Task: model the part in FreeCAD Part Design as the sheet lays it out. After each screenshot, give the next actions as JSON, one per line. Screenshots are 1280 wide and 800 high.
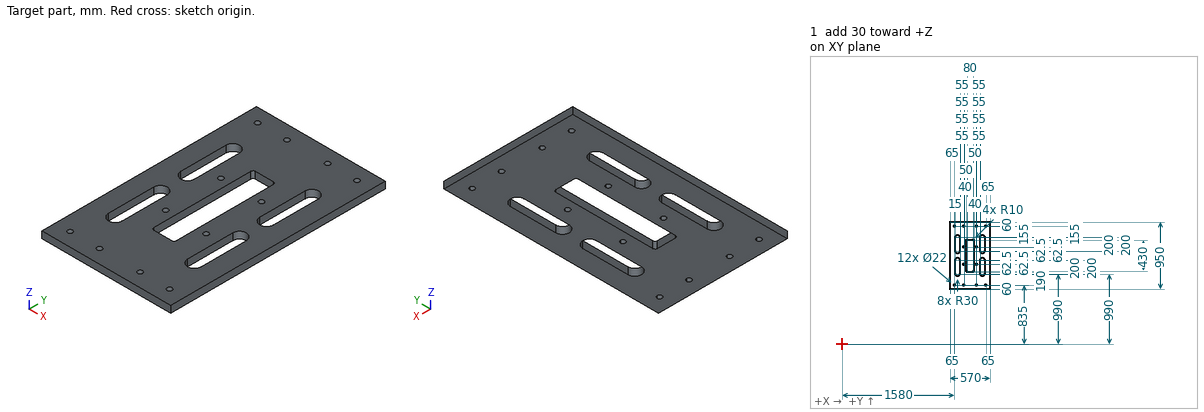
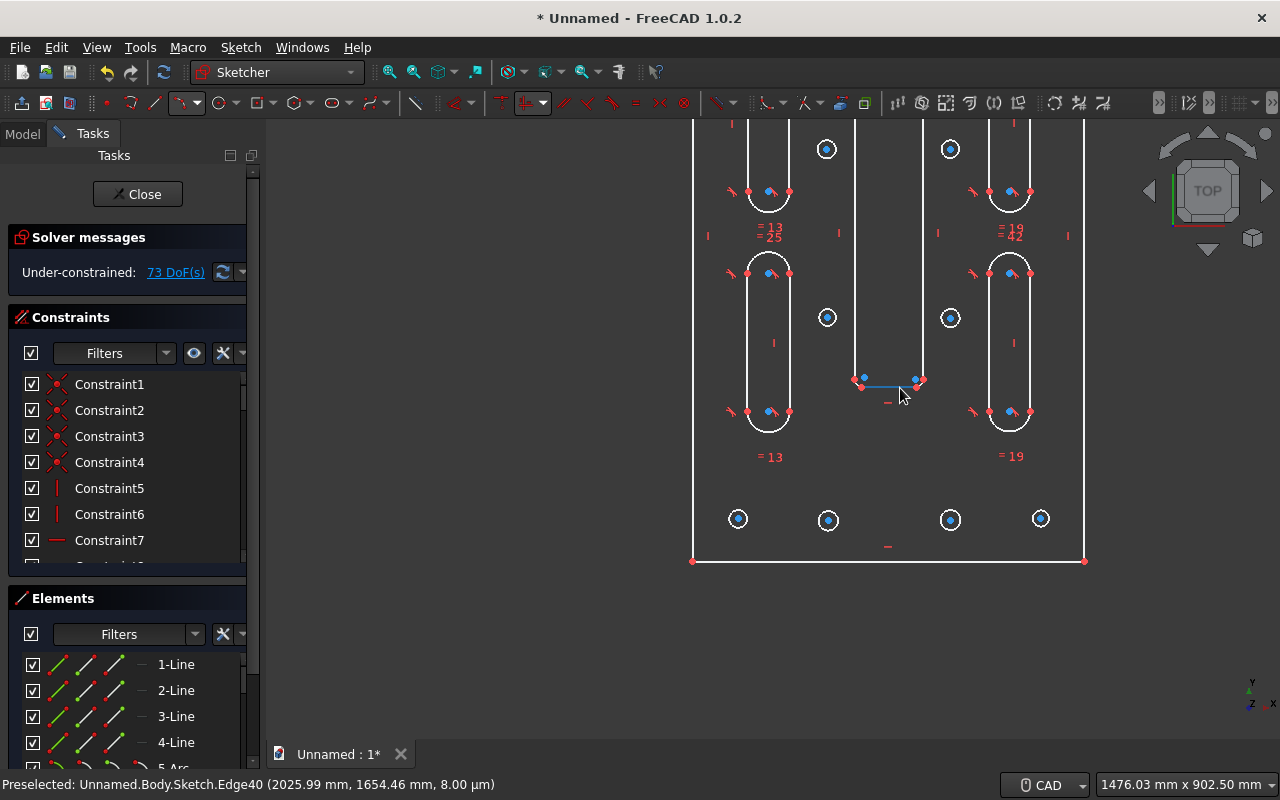
{"action": "left_click", "coordinate": [900, 387]}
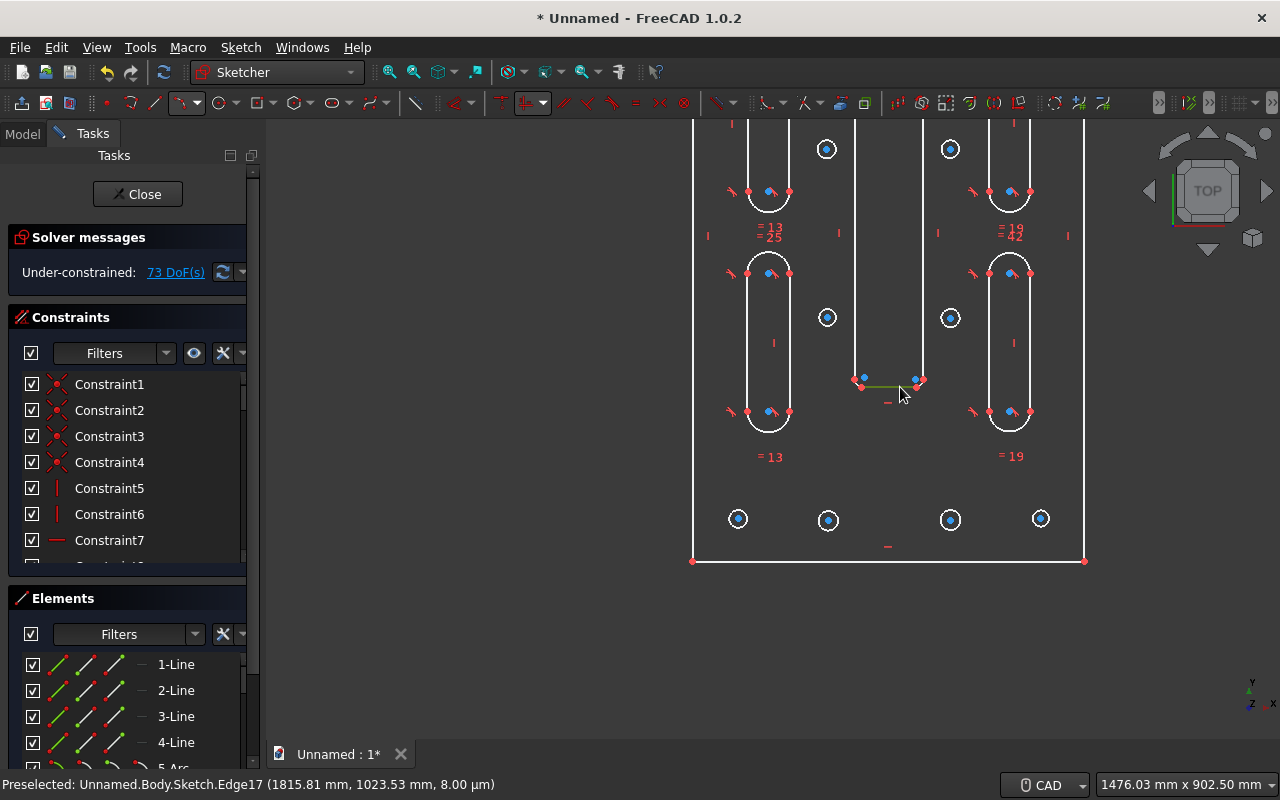
{"action": "scroll", "coordinate": [857, 385], "scroll_direction": "up", "scroll_amount": 5}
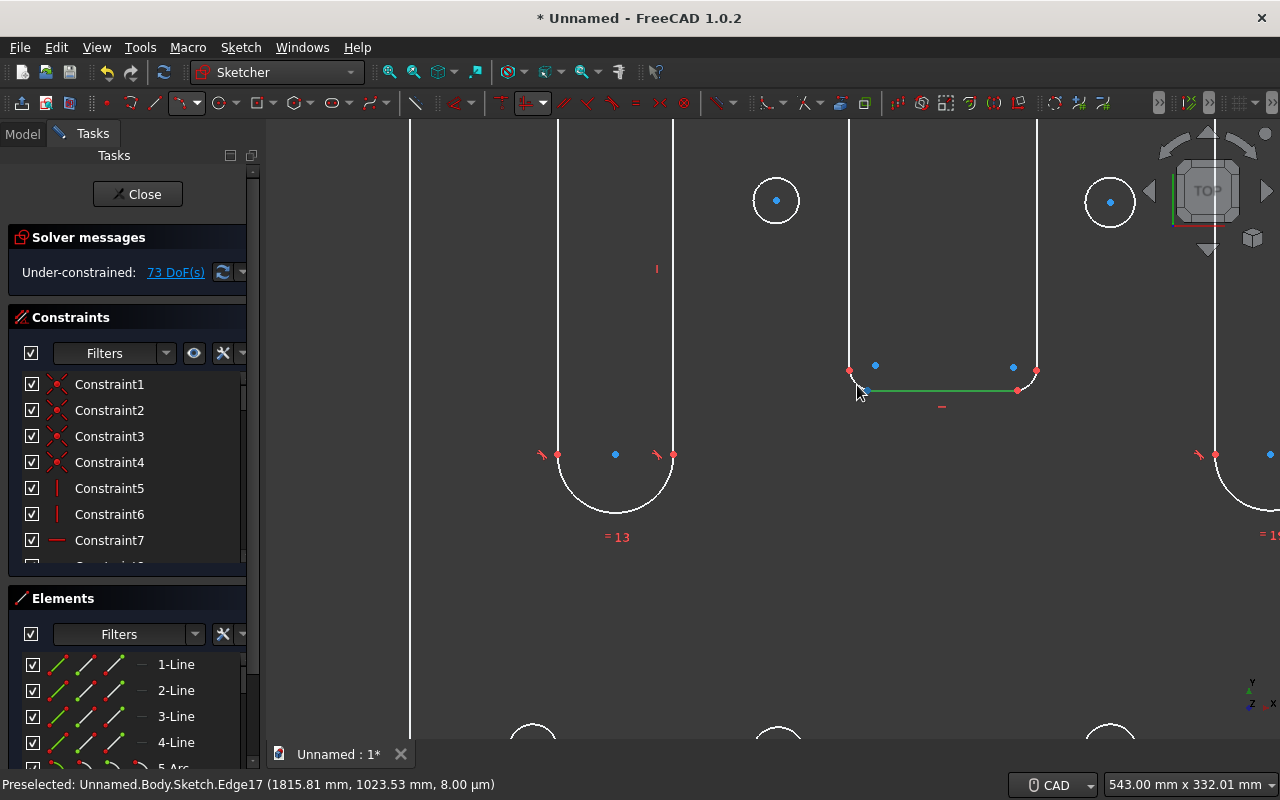
{"action": "left_click", "coordinate": [856, 383]}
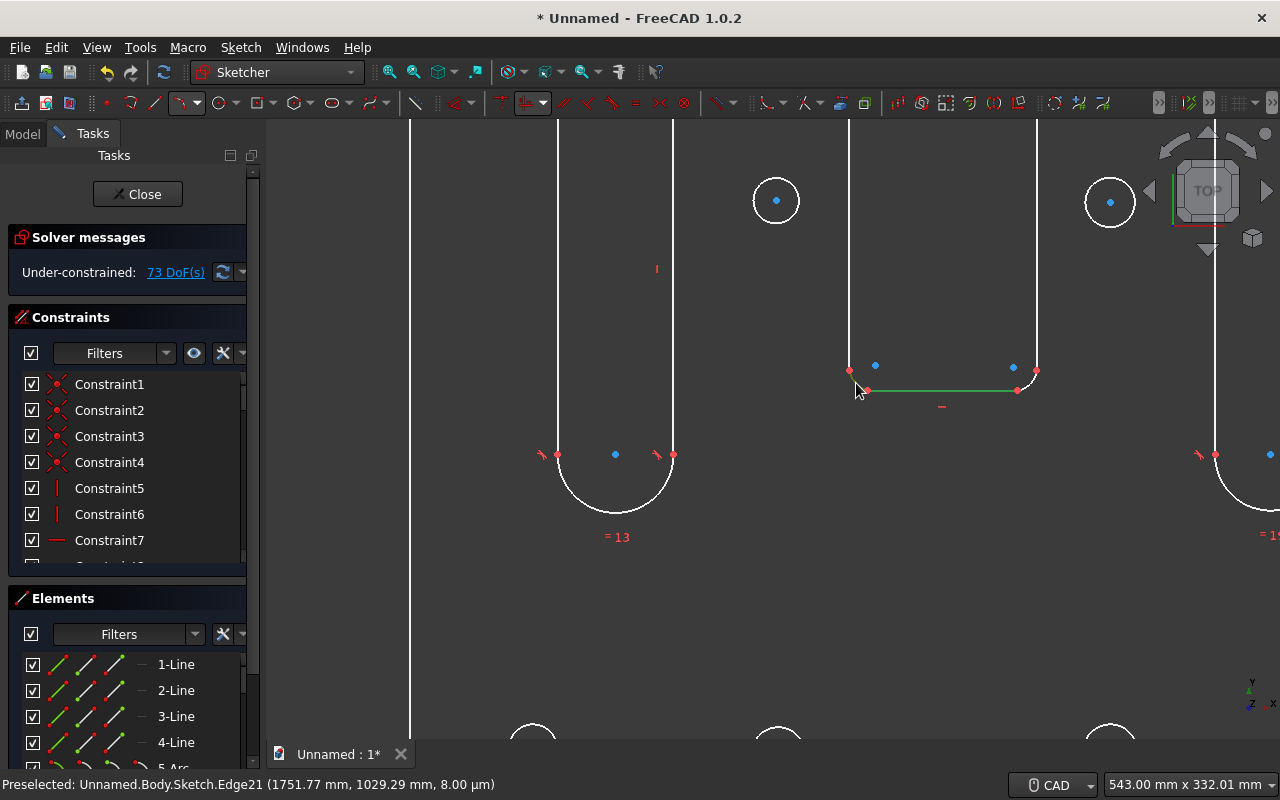
{"action": "key", "text": "t"}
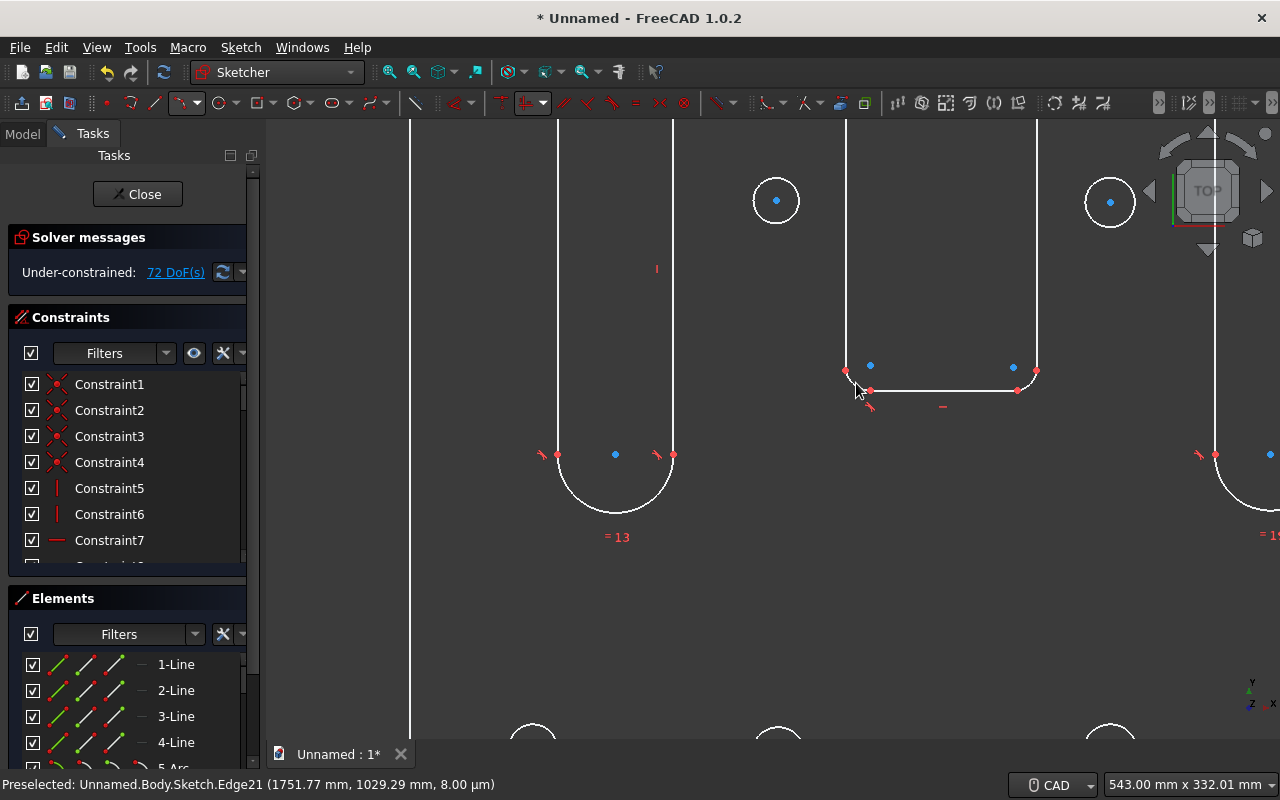
{"action": "scroll", "coordinate": [889, 388], "scroll_direction": "down", "scroll_amount": 10}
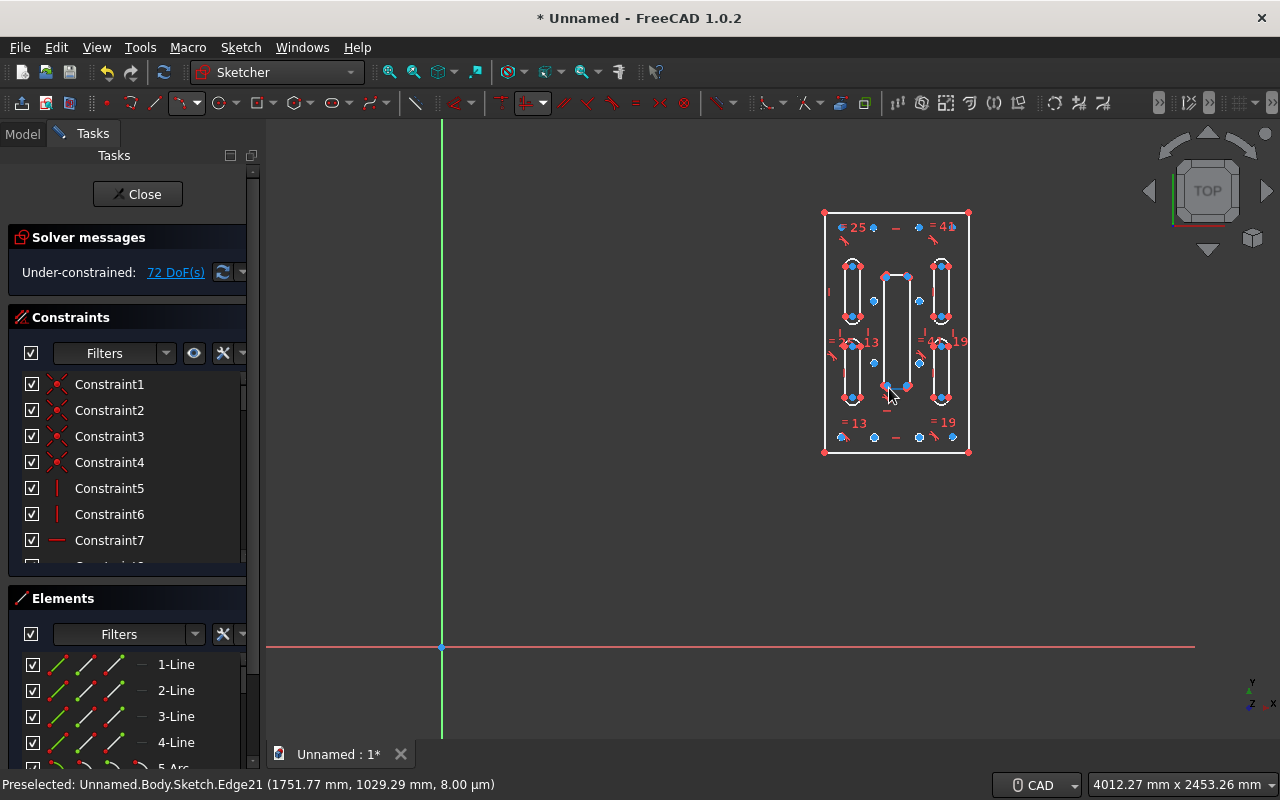
{"action": "scroll", "coordinate": [901, 389], "scroll_direction": "up", "scroll_amount": 5}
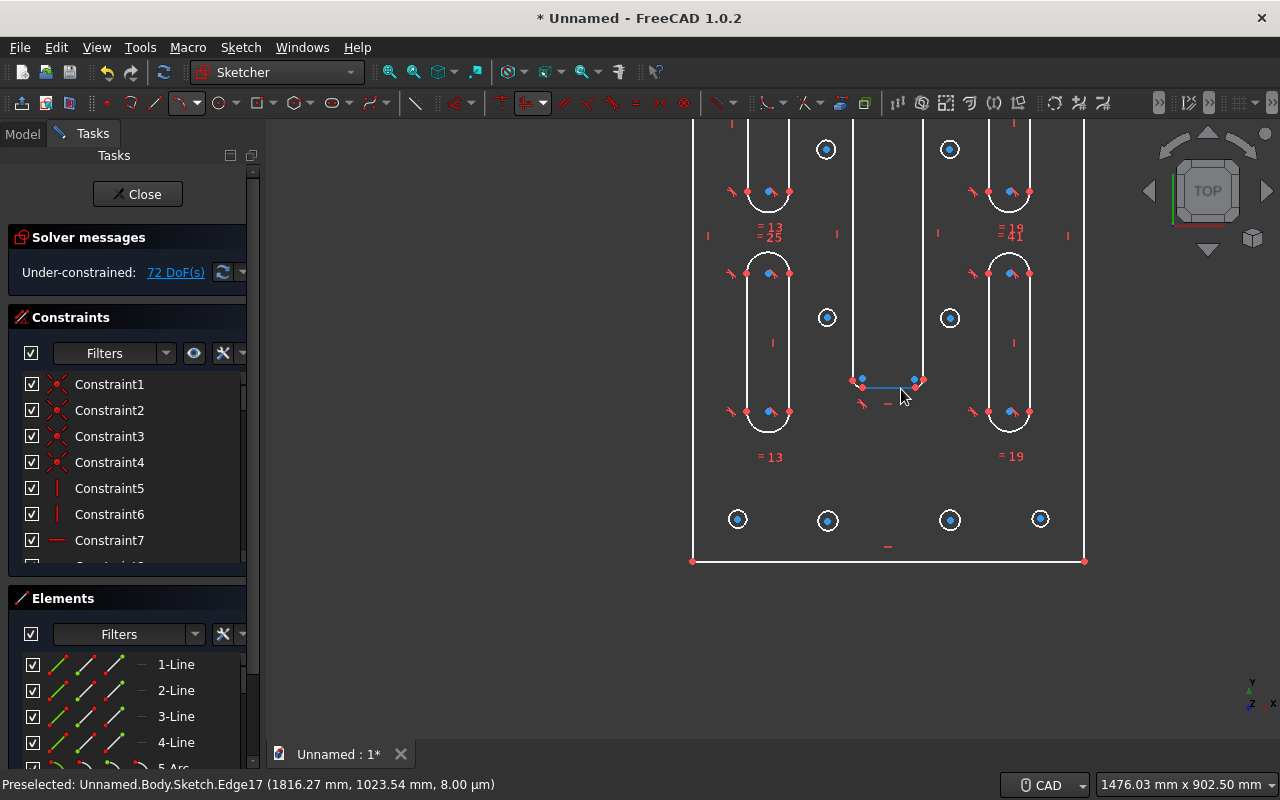
{"action": "left_click", "coordinate": [900, 388]}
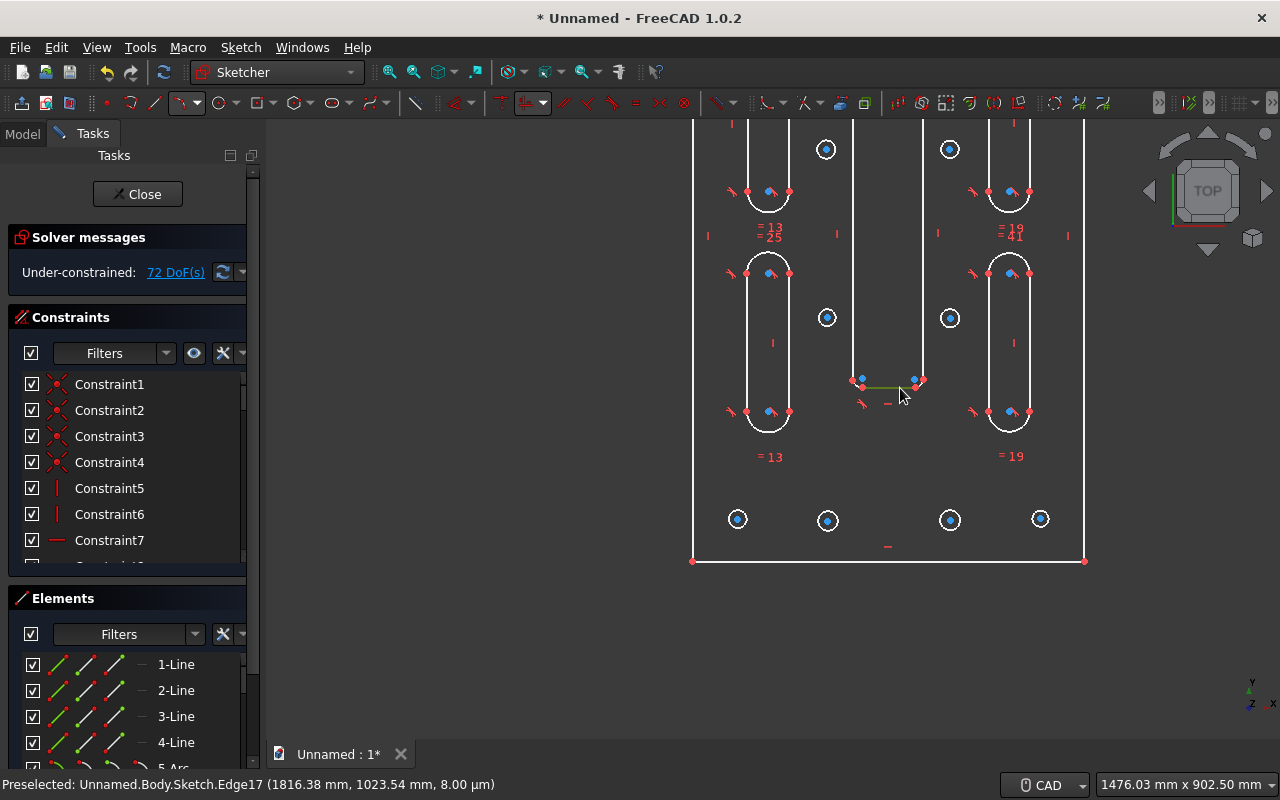
{"action": "scroll", "coordinate": [921, 385], "scroll_direction": "up", "scroll_amount": 5}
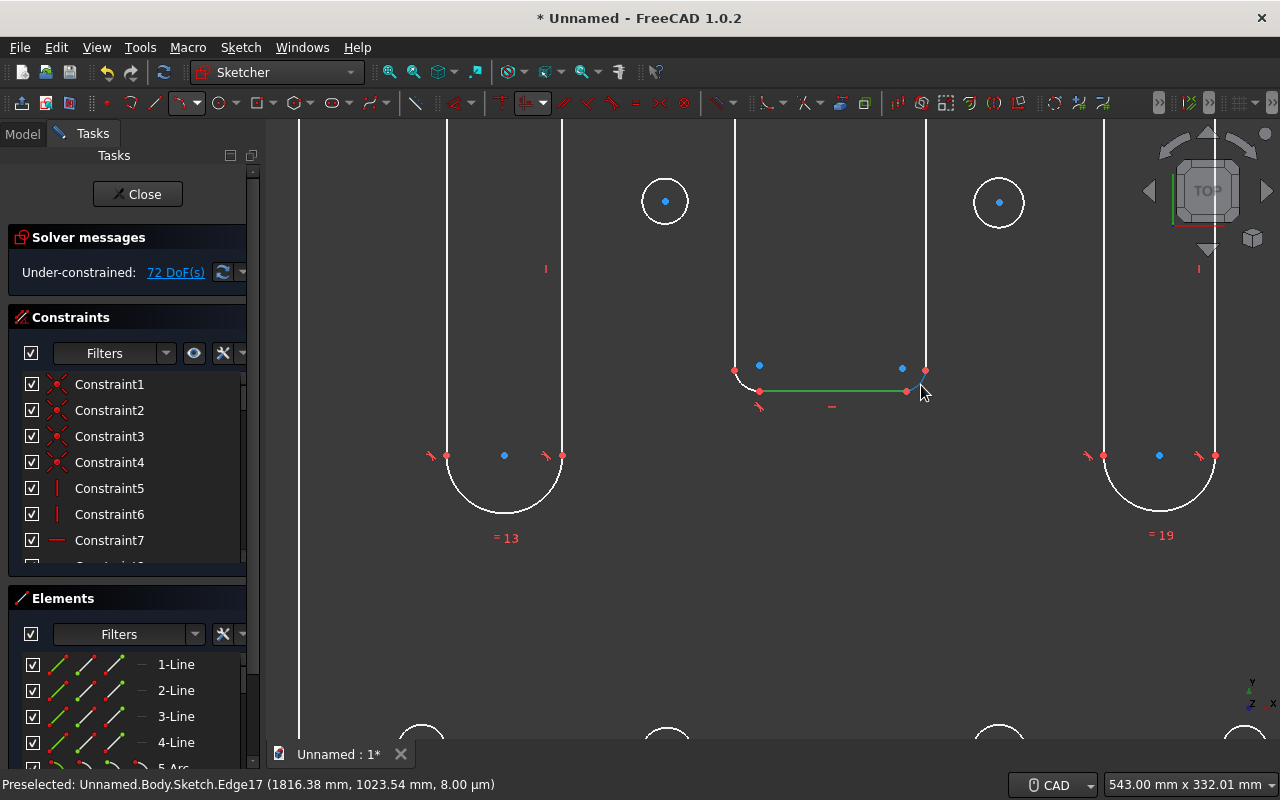
{"action": "left_click", "coordinate": [919, 384]}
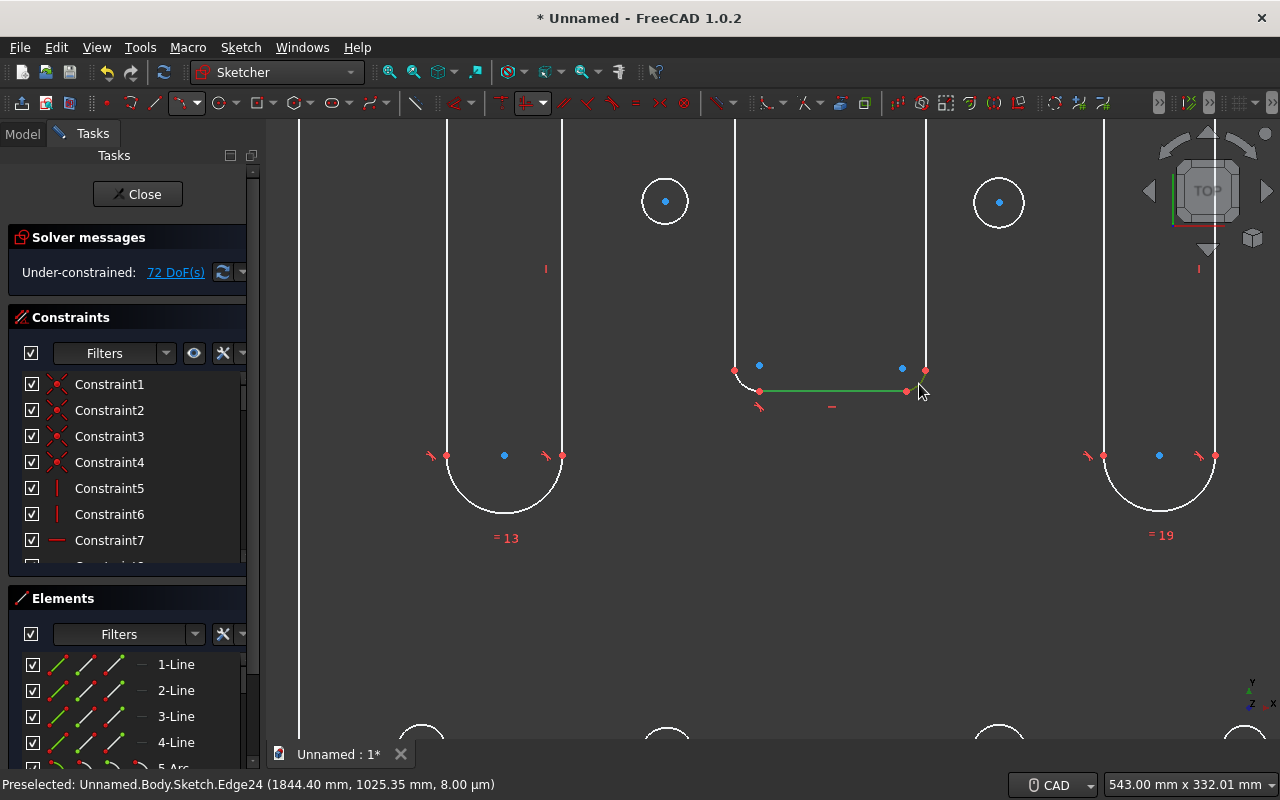
{"action": "key", "text": "t"}